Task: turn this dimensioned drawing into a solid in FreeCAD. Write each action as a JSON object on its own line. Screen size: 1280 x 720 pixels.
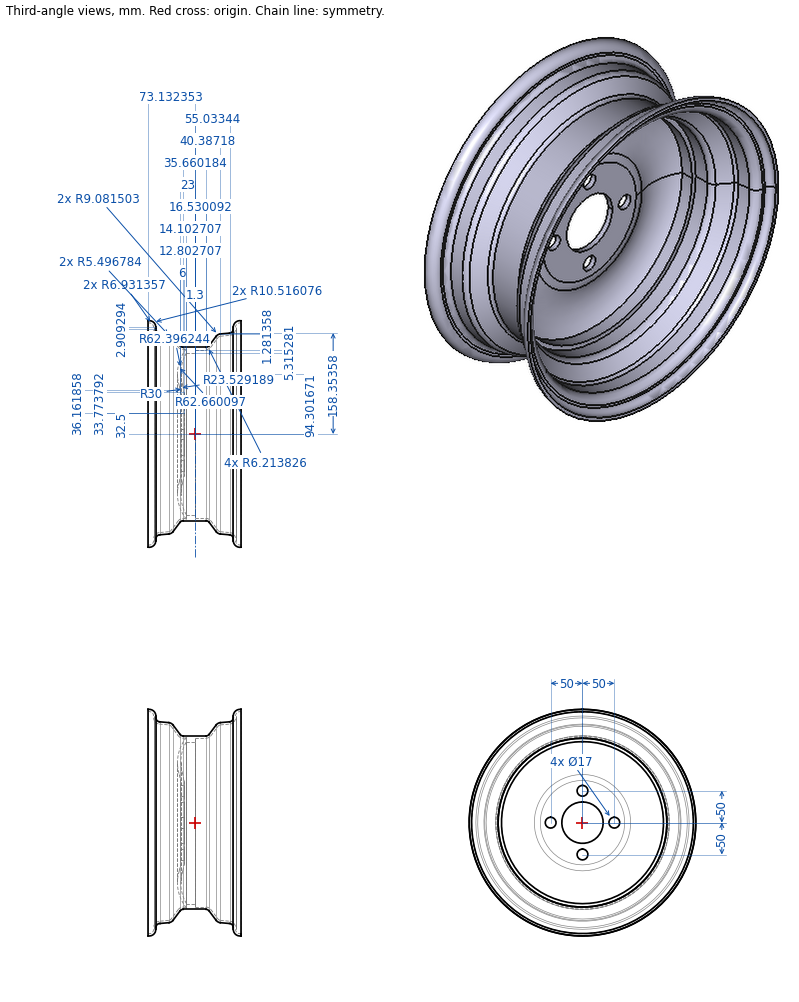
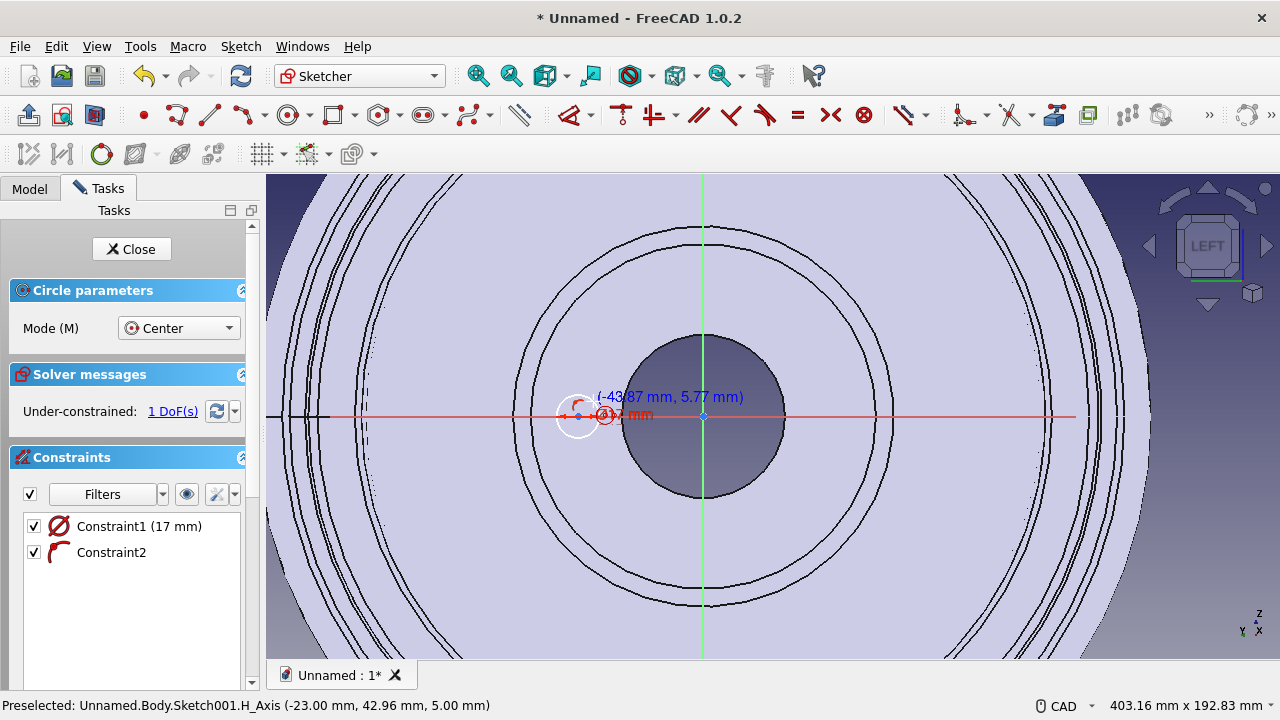
{"action": "left_click", "coordinate": [703, 291]}
{"action": "mouse_move", "coordinate": [718, 276]}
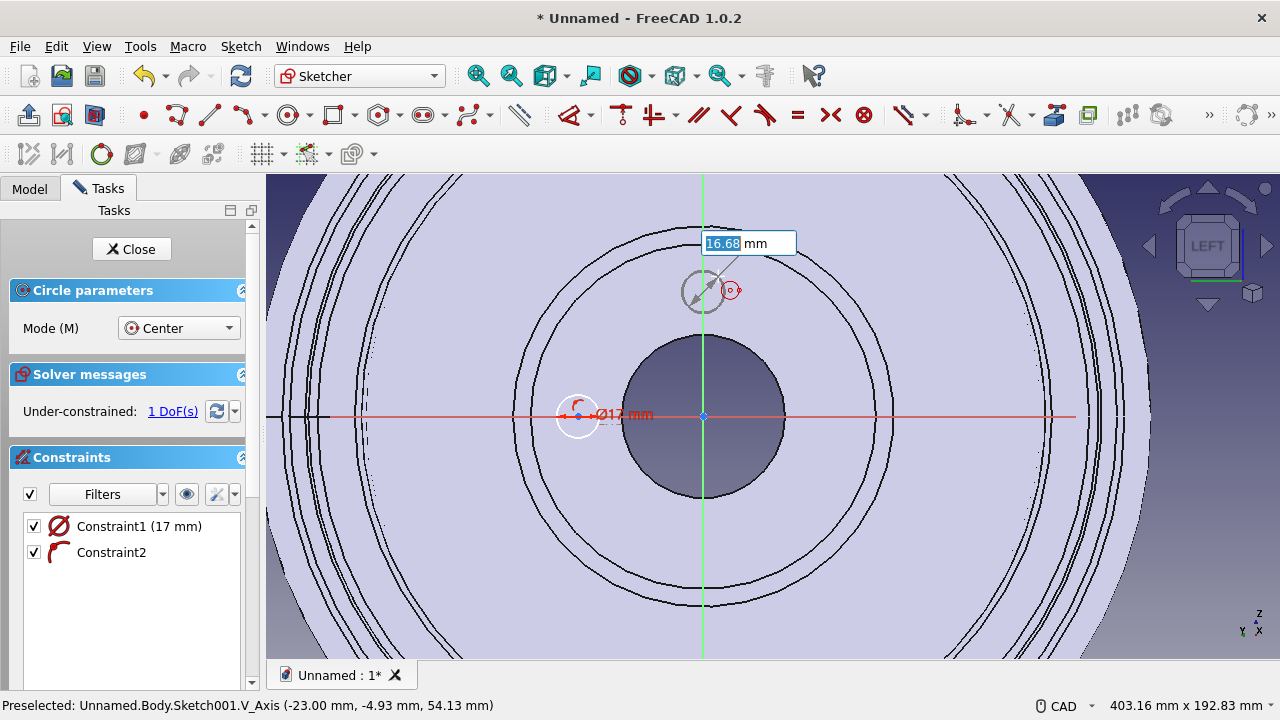
{"action": "type", "text": "17"}
{"action": "key", "text": "Return"}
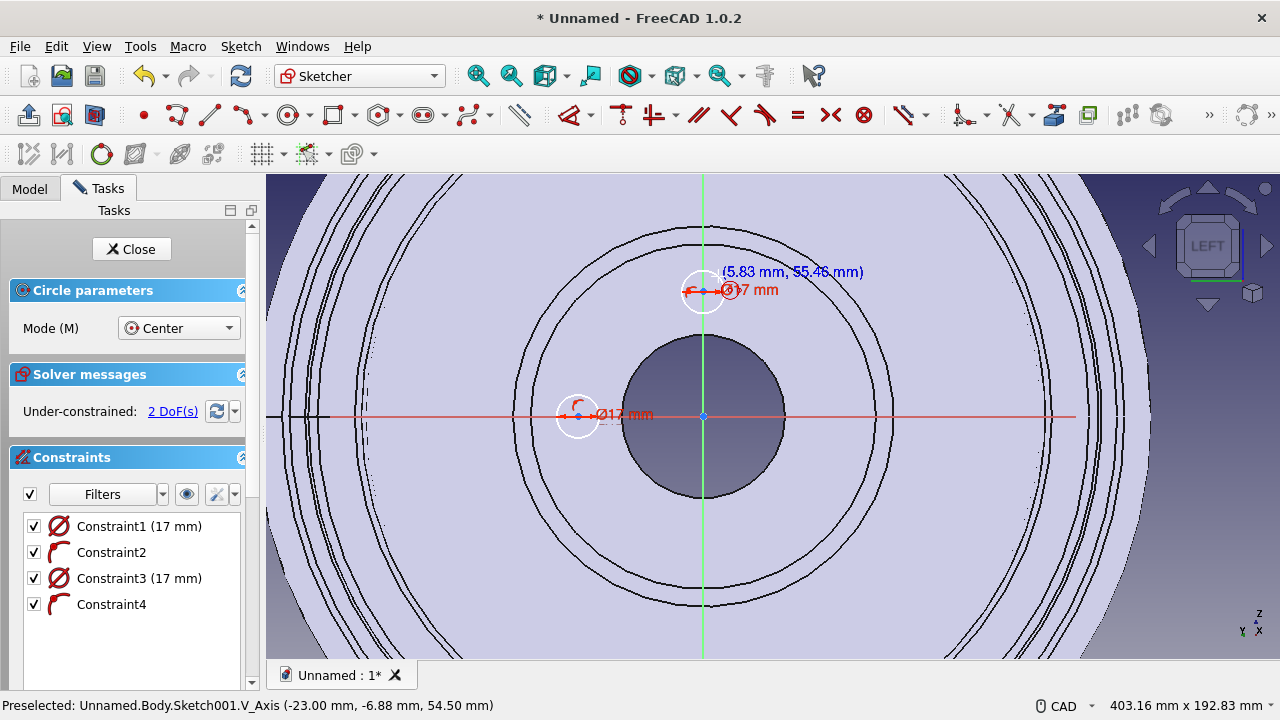
{"action": "left_click", "coordinate": [829, 416]}
{"action": "mouse_move", "coordinate": [844, 401]}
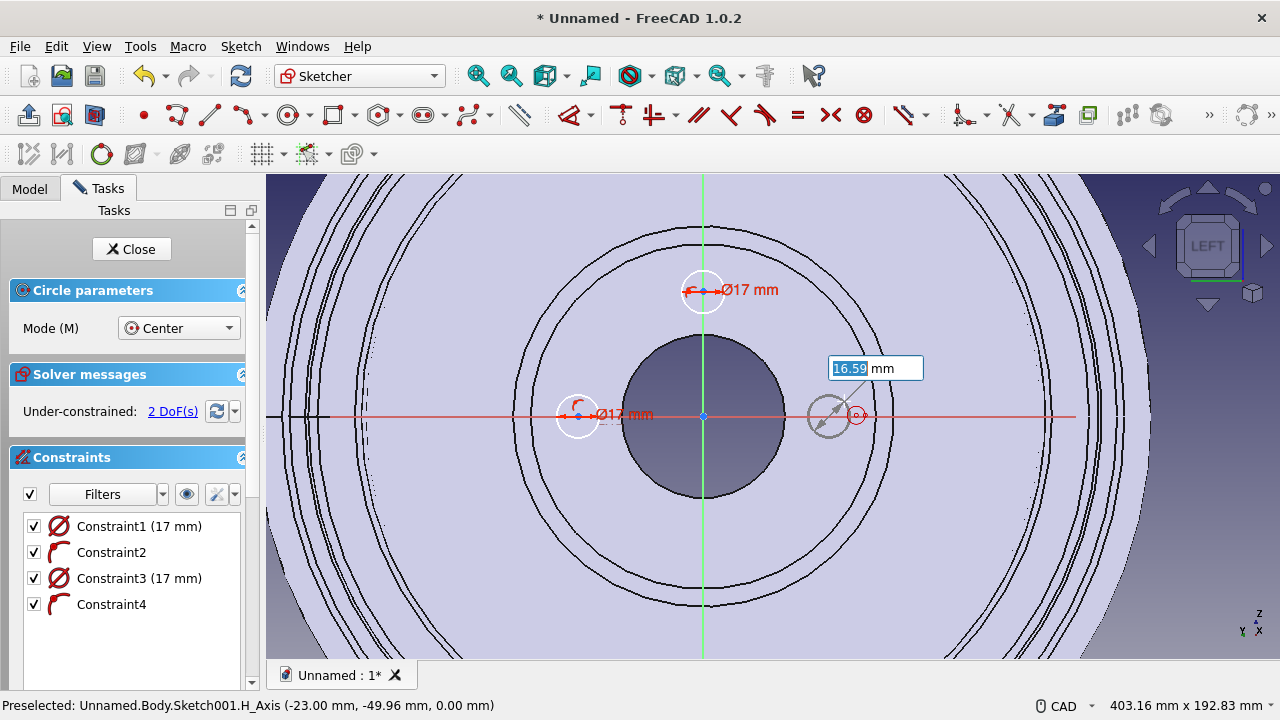
{"action": "type", "text": "17"}
{"action": "key", "text": "Return"}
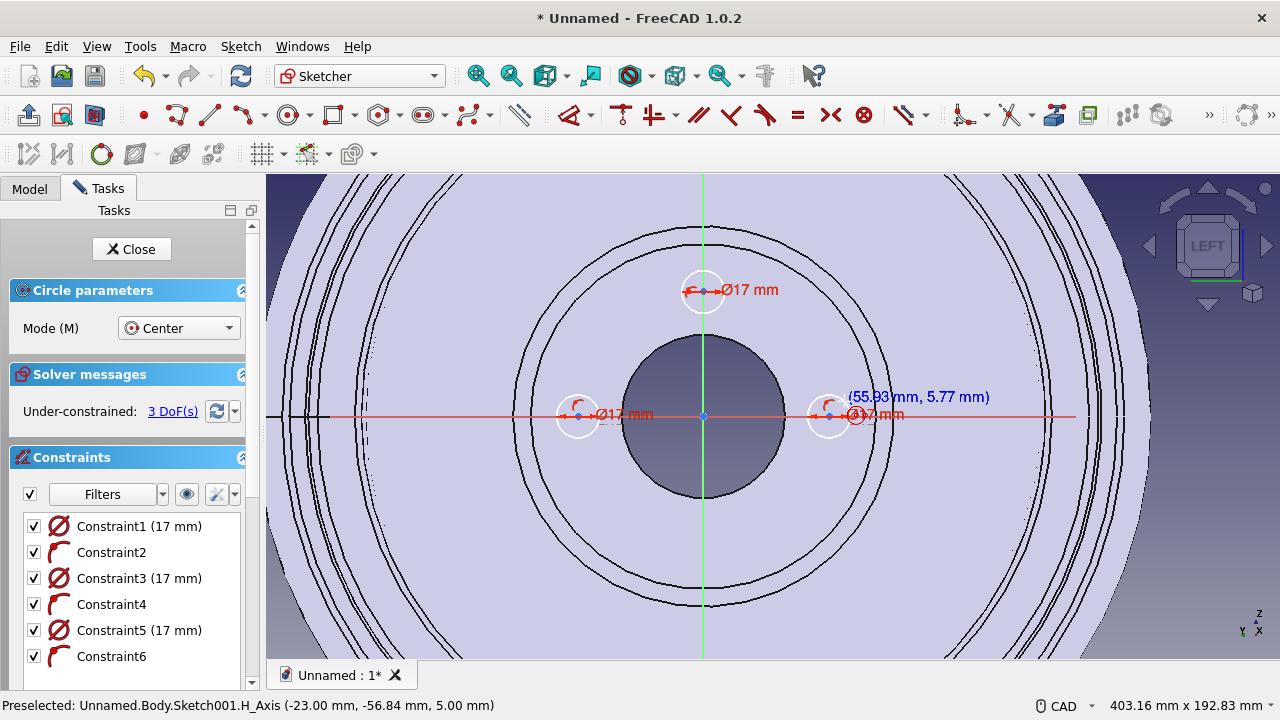
{"action": "left_click", "coordinate": [703, 542]}
{"action": "mouse_move", "coordinate": [718, 527]}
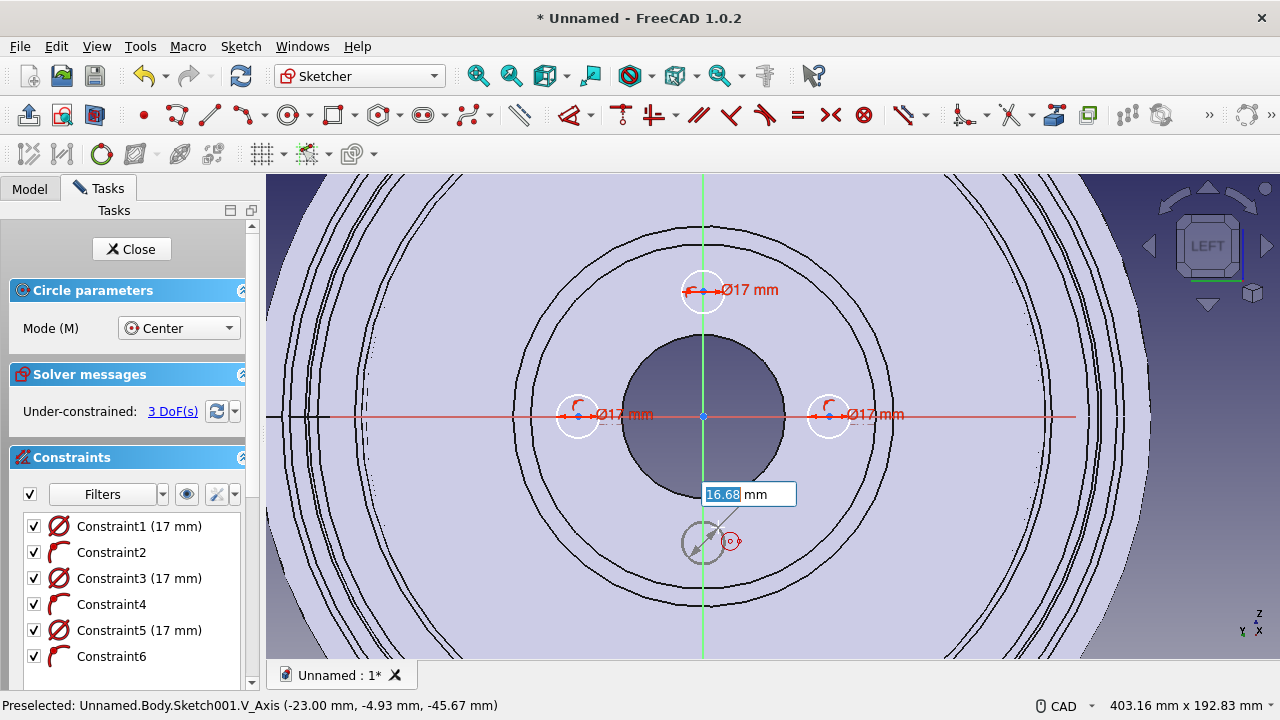
{"action": "type", "text": "17"}
{"action": "key", "text": "Return"}
{"action": "key", "text": "Escape"}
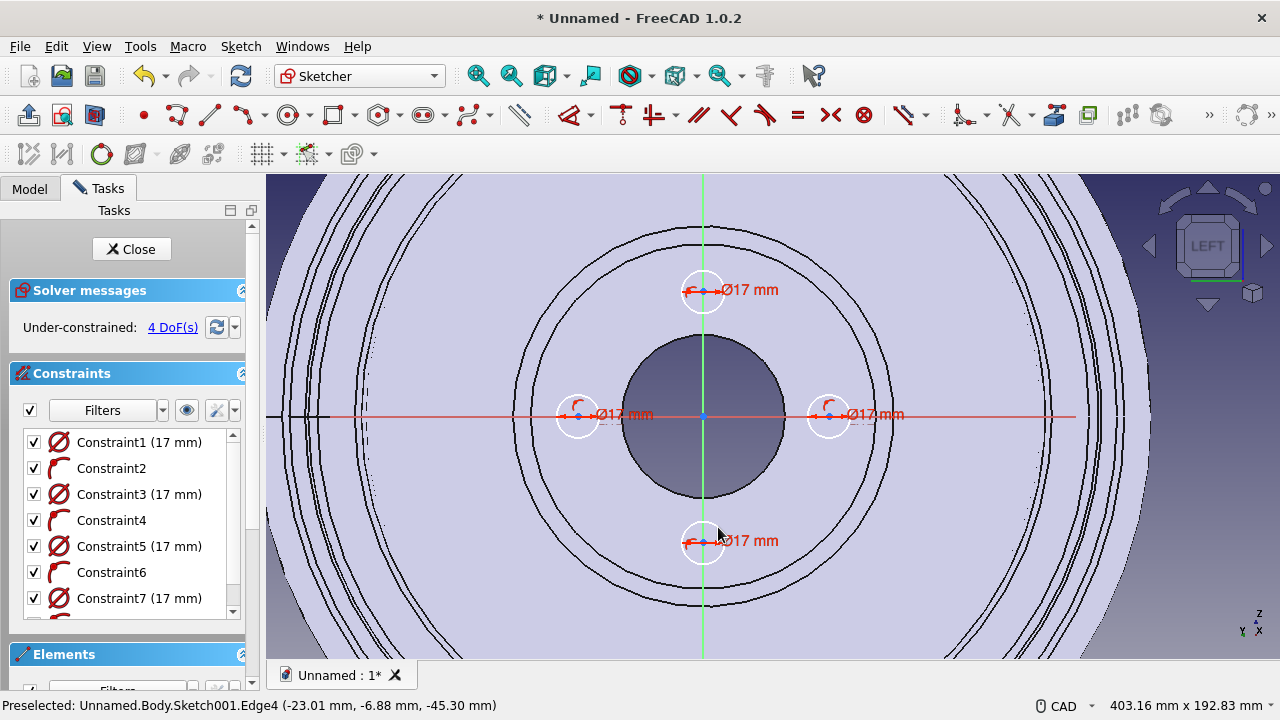
{"action": "key", "text": "d"}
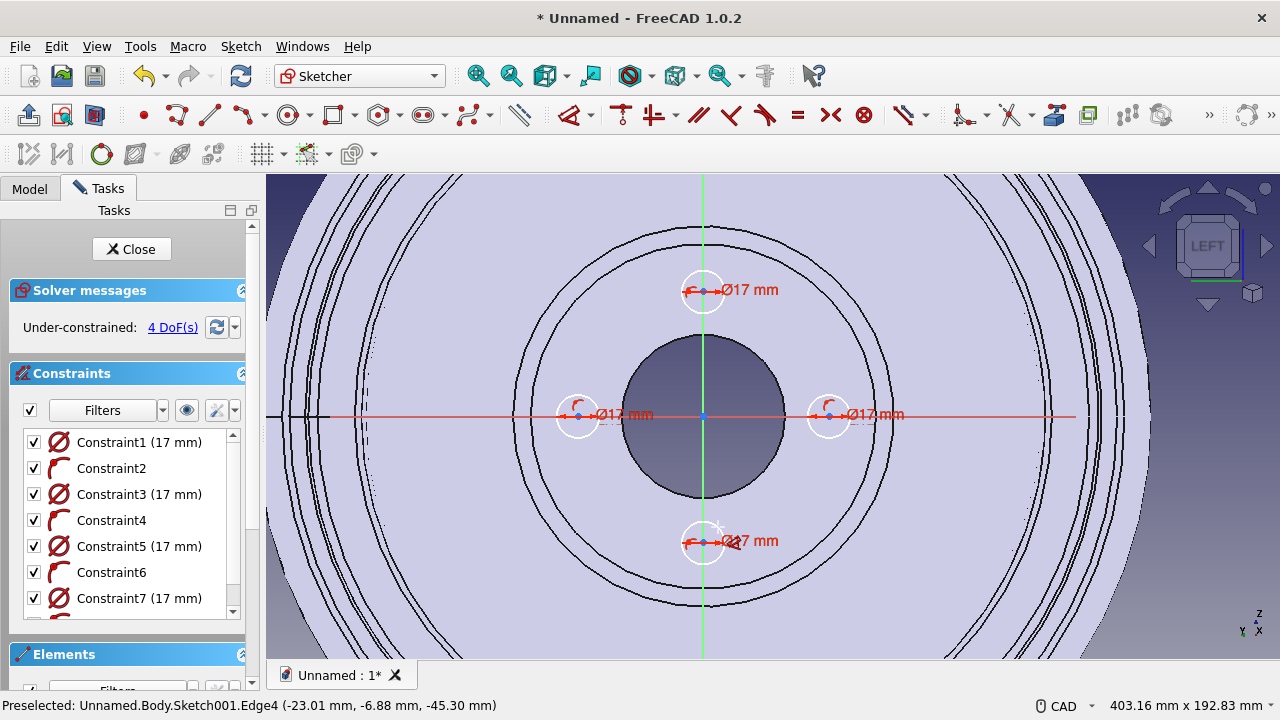
{"action": "left_click", "coordinate": [578, 416]}
{"action": "left_click", "coordinate": [641, 450]}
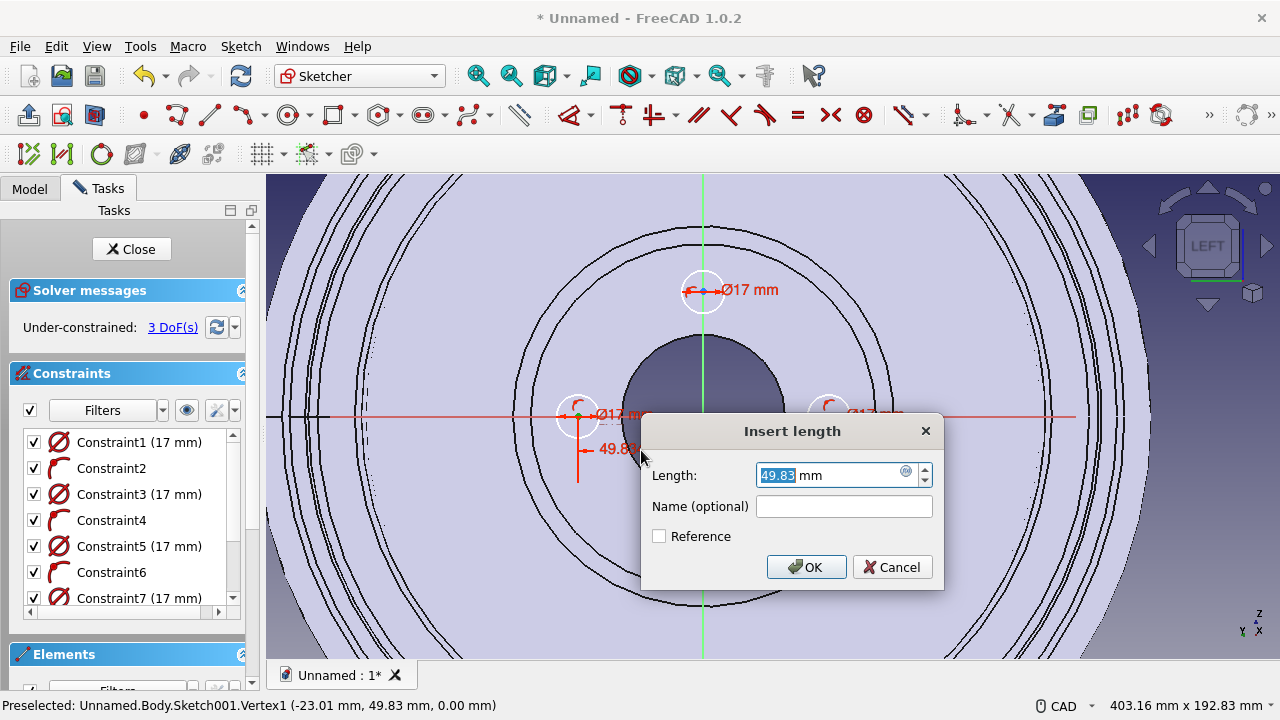
{"action": "type", "text": "50"}
{"action": "key", "text": "Return"}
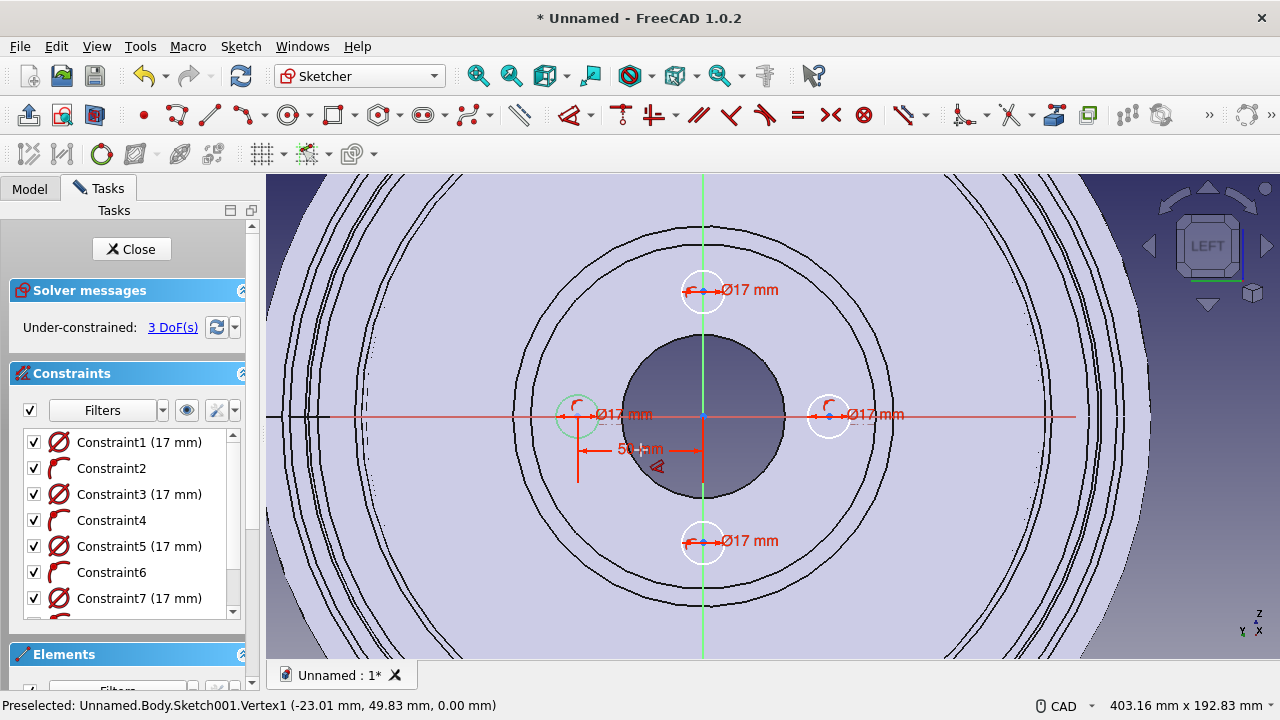
{"action": "left_click", "coordinate": [703, 292]}
{"action": "left_click", "coordinate": [737, 354]}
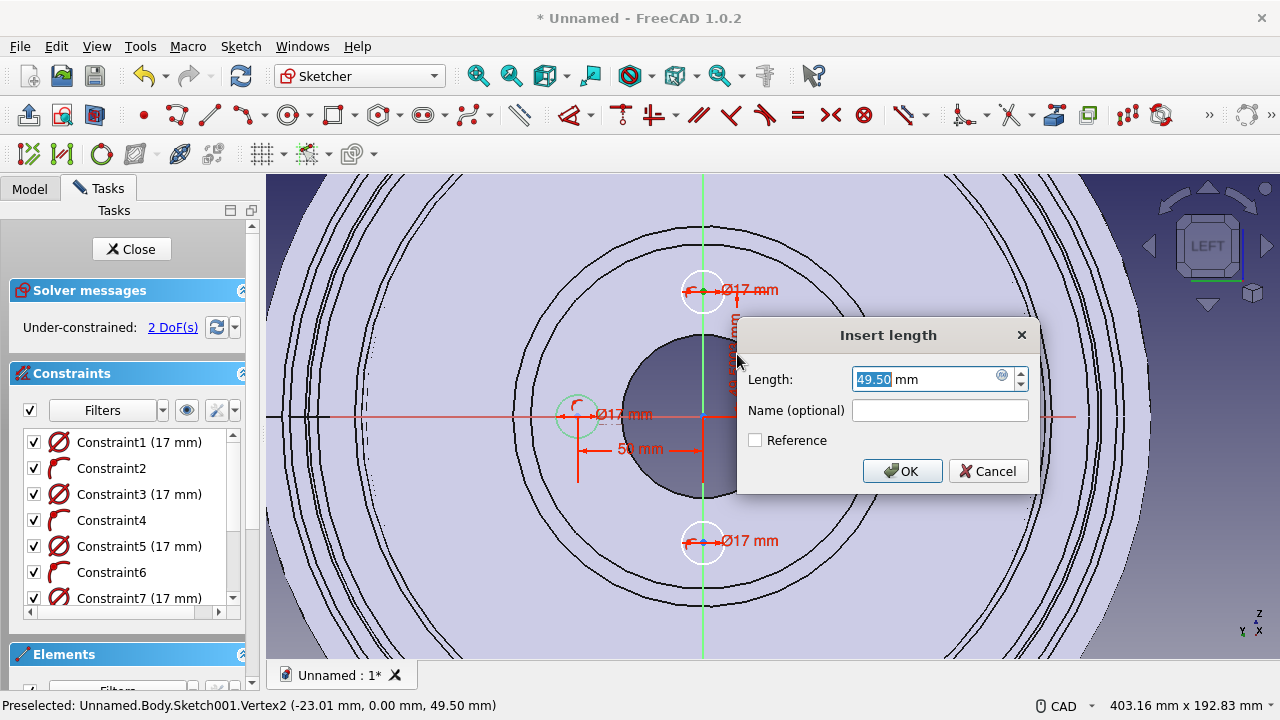
{"action": "type", "text": "50"}
{"action": "key", "text": "Return"}